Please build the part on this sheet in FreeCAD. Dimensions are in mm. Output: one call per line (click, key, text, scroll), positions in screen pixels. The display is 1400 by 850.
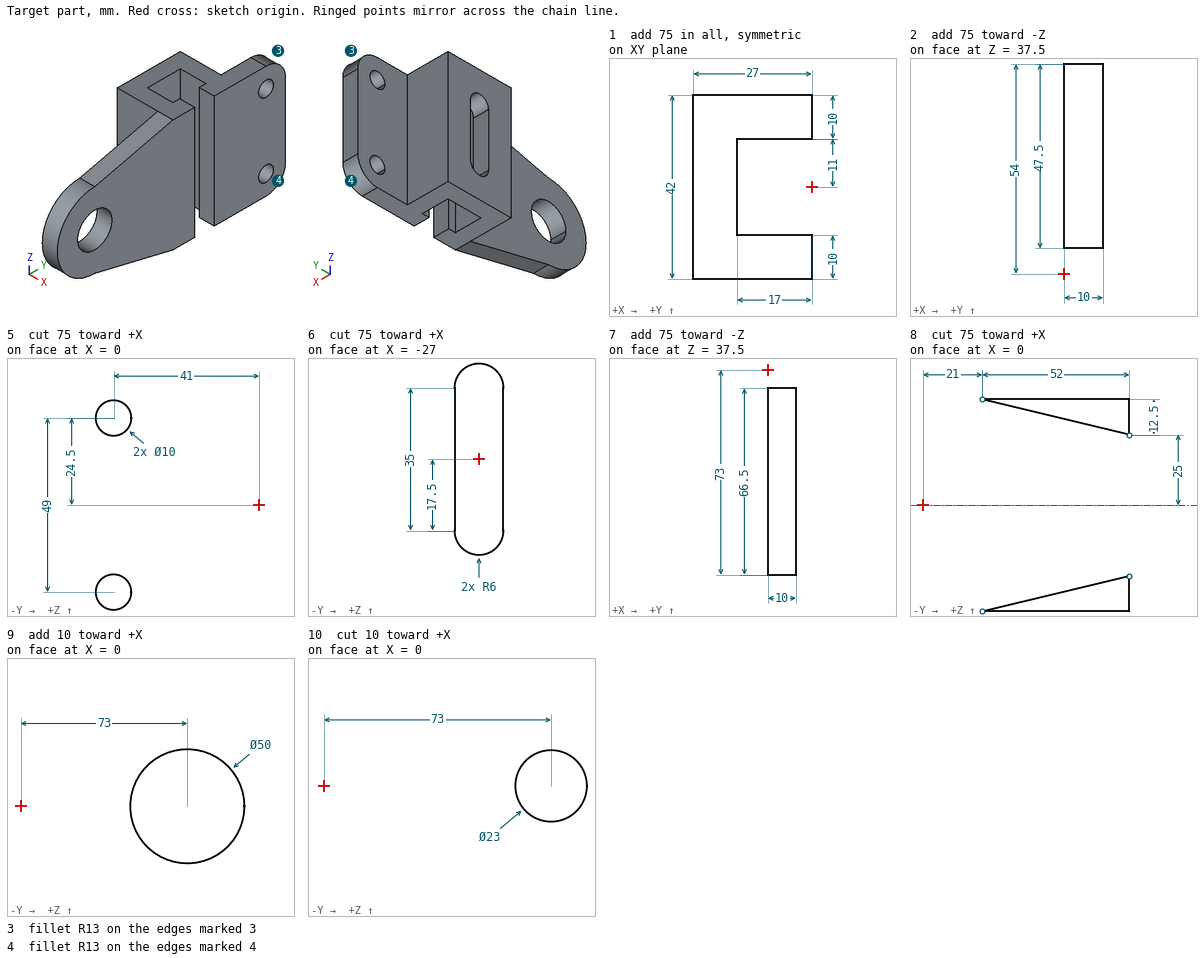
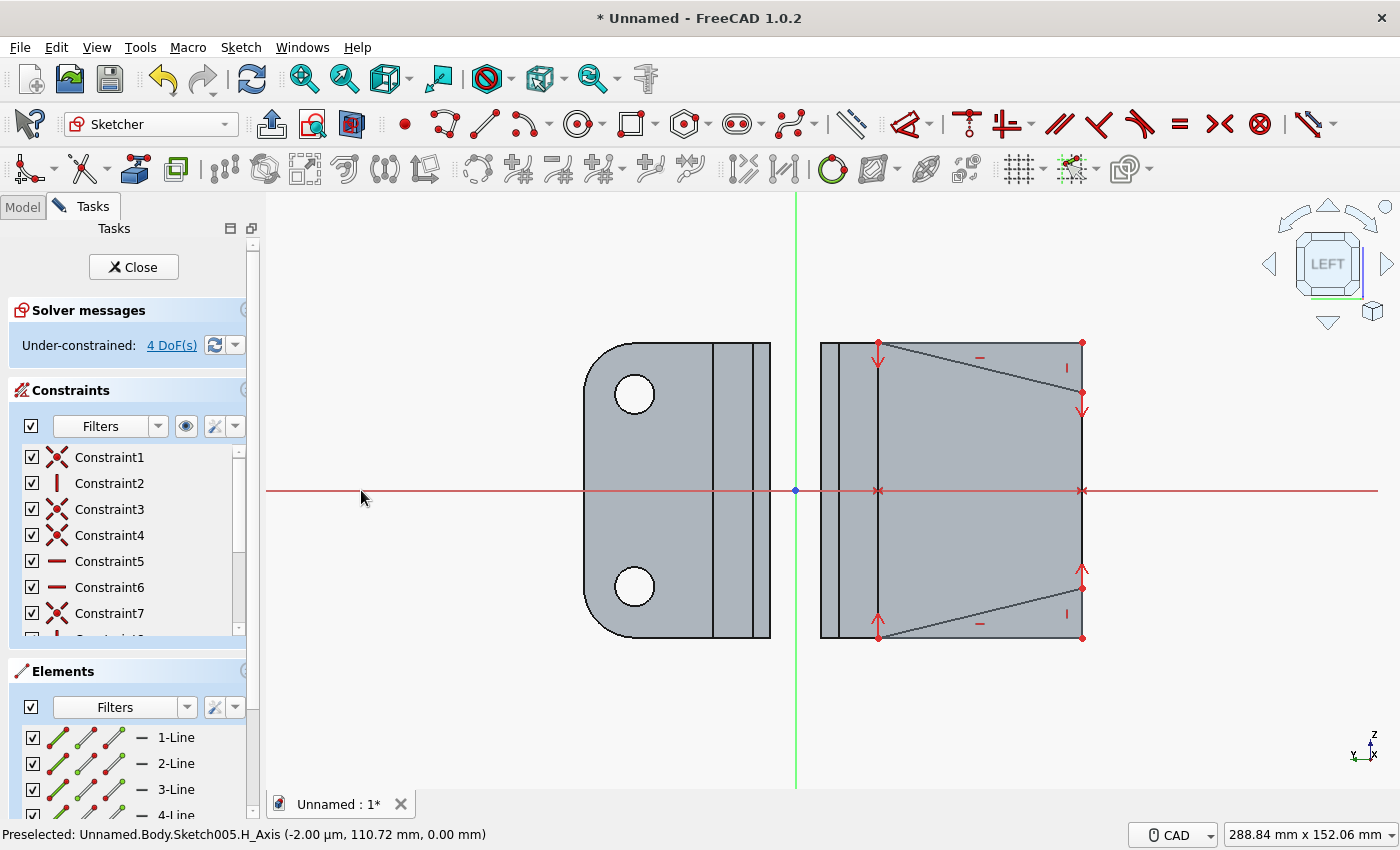
click(1021, 343)
click(980, 309)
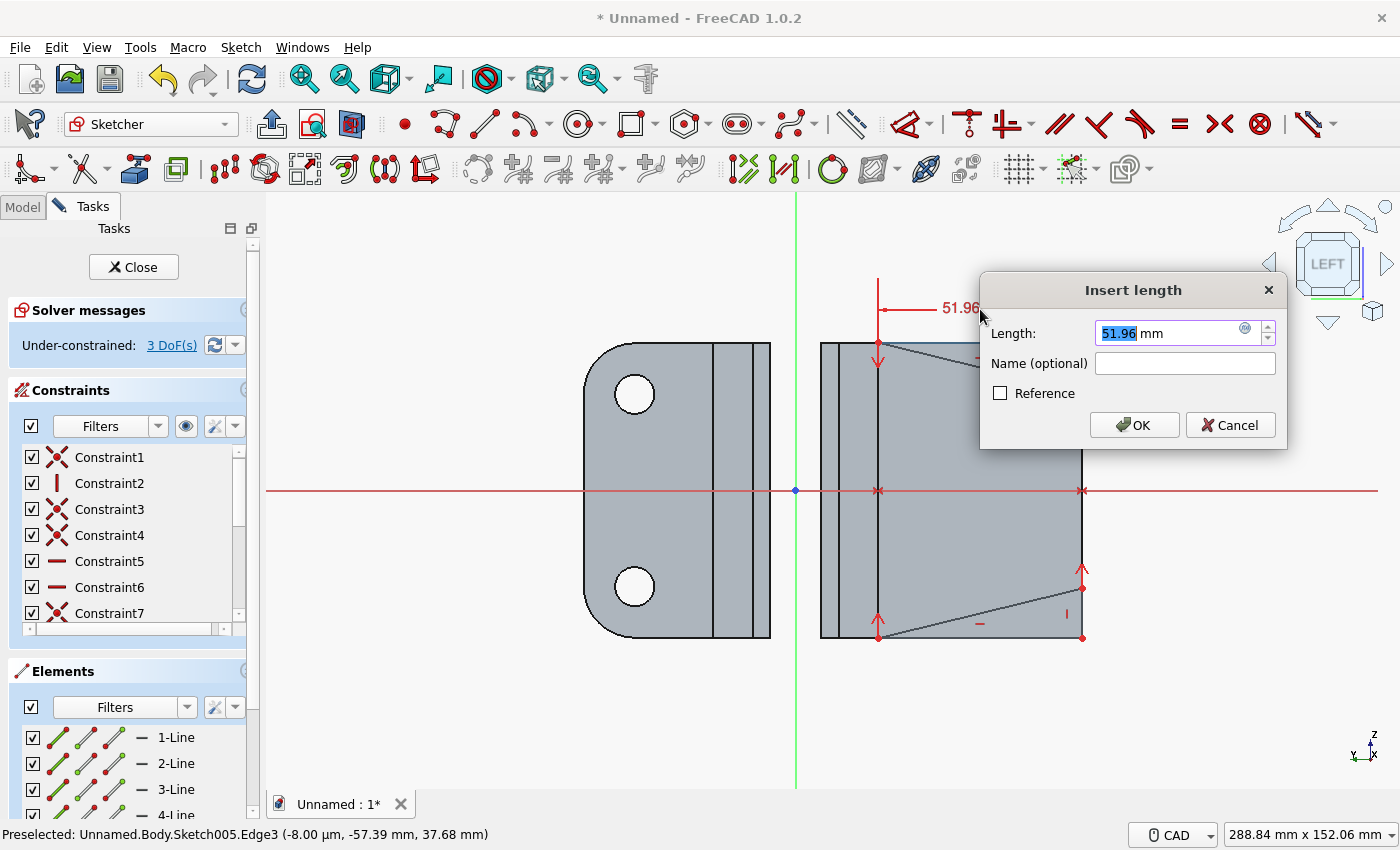
text(52)
key(Return)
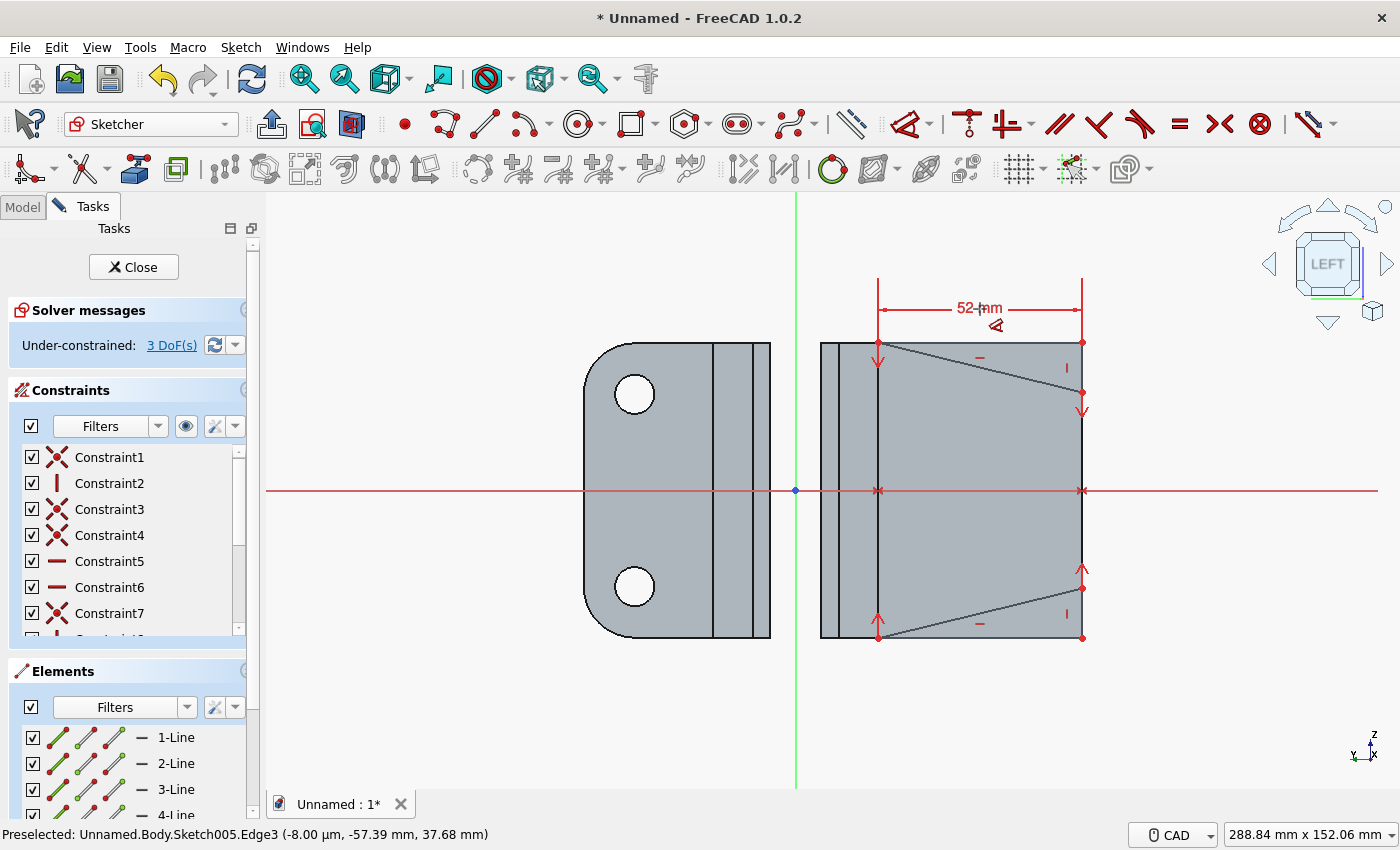
click(878, 343)
click(837, 309)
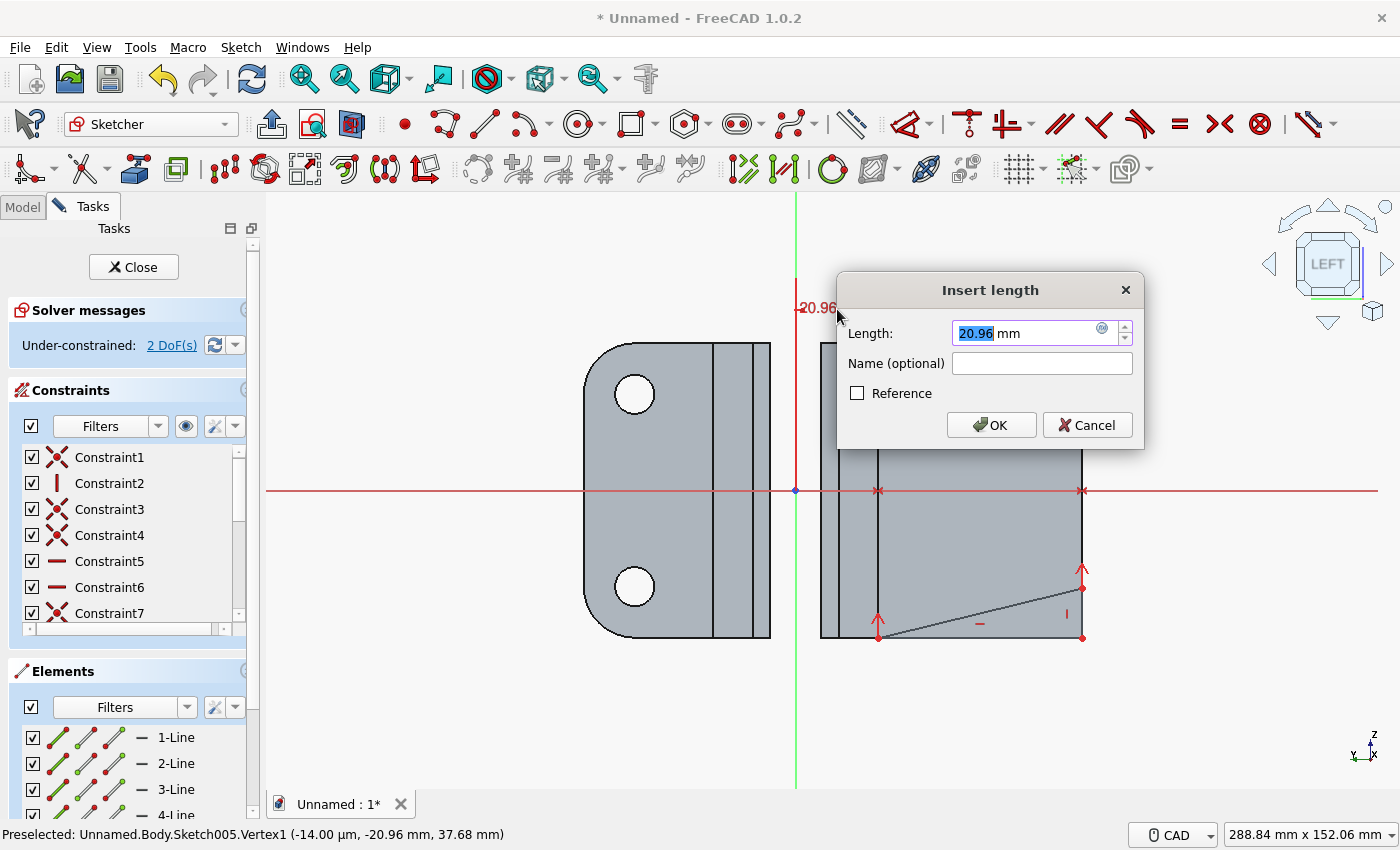
text(21)
key(Return)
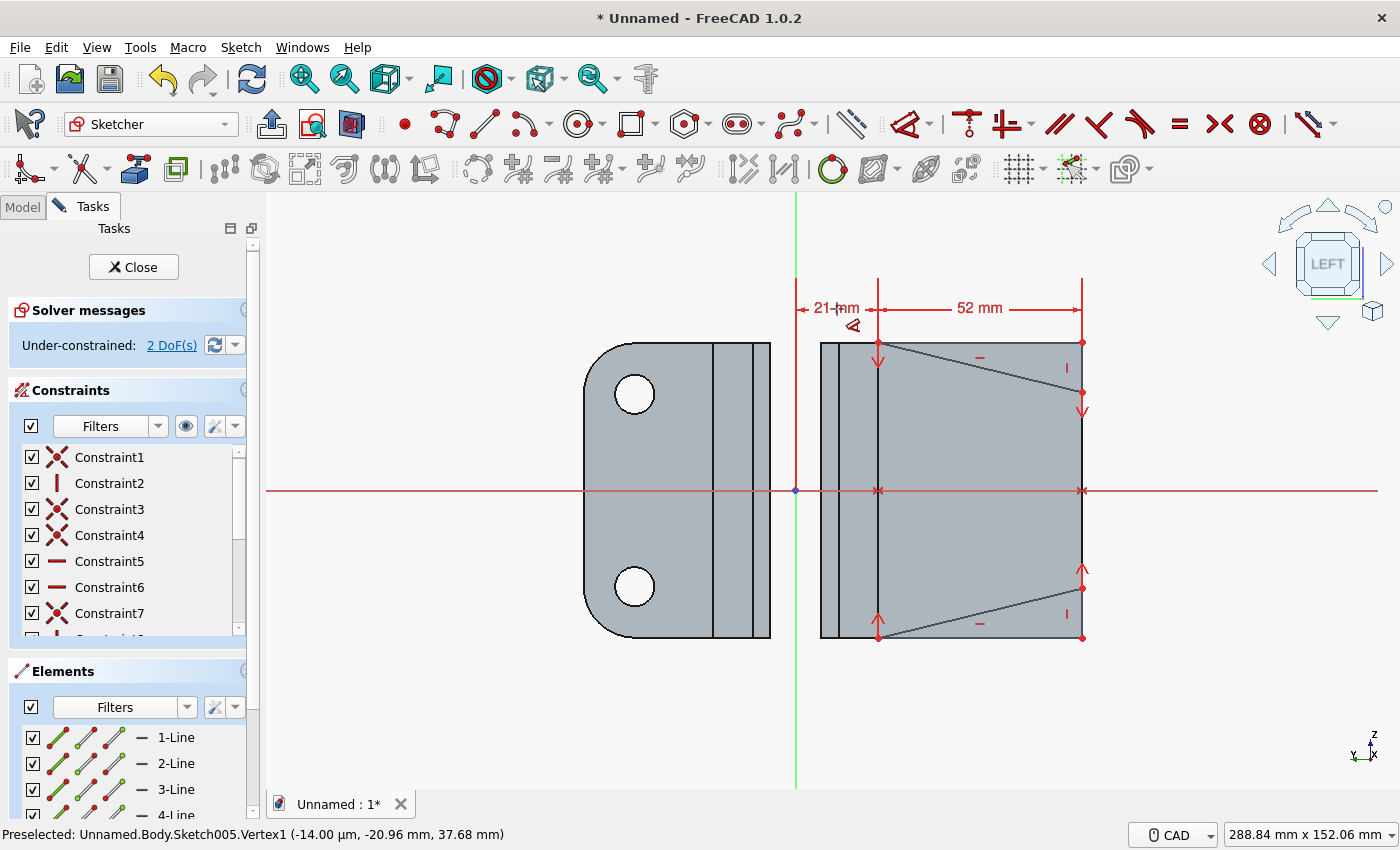
click(1082, 392)
click(1116, 441)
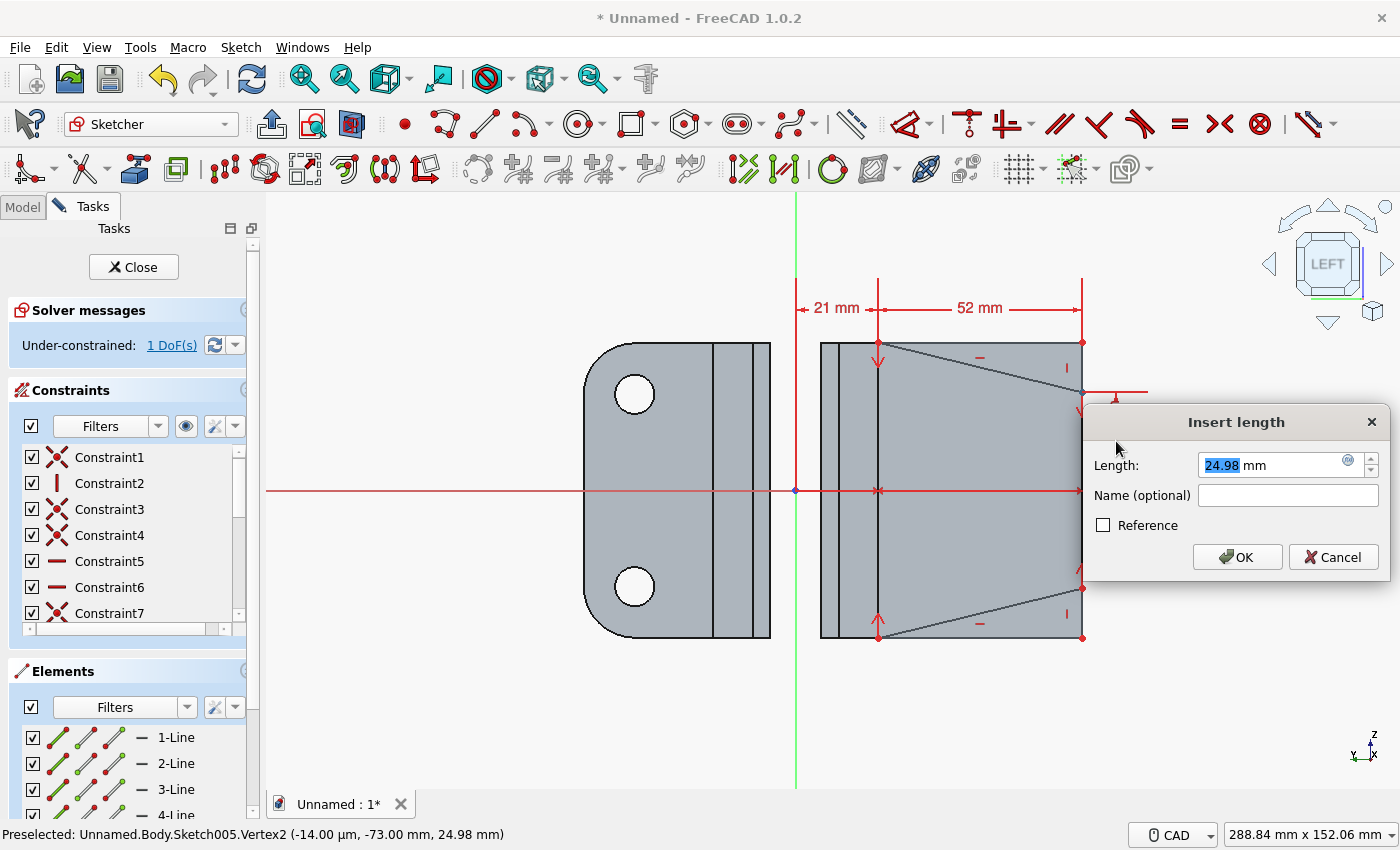
text(25)
key(Return)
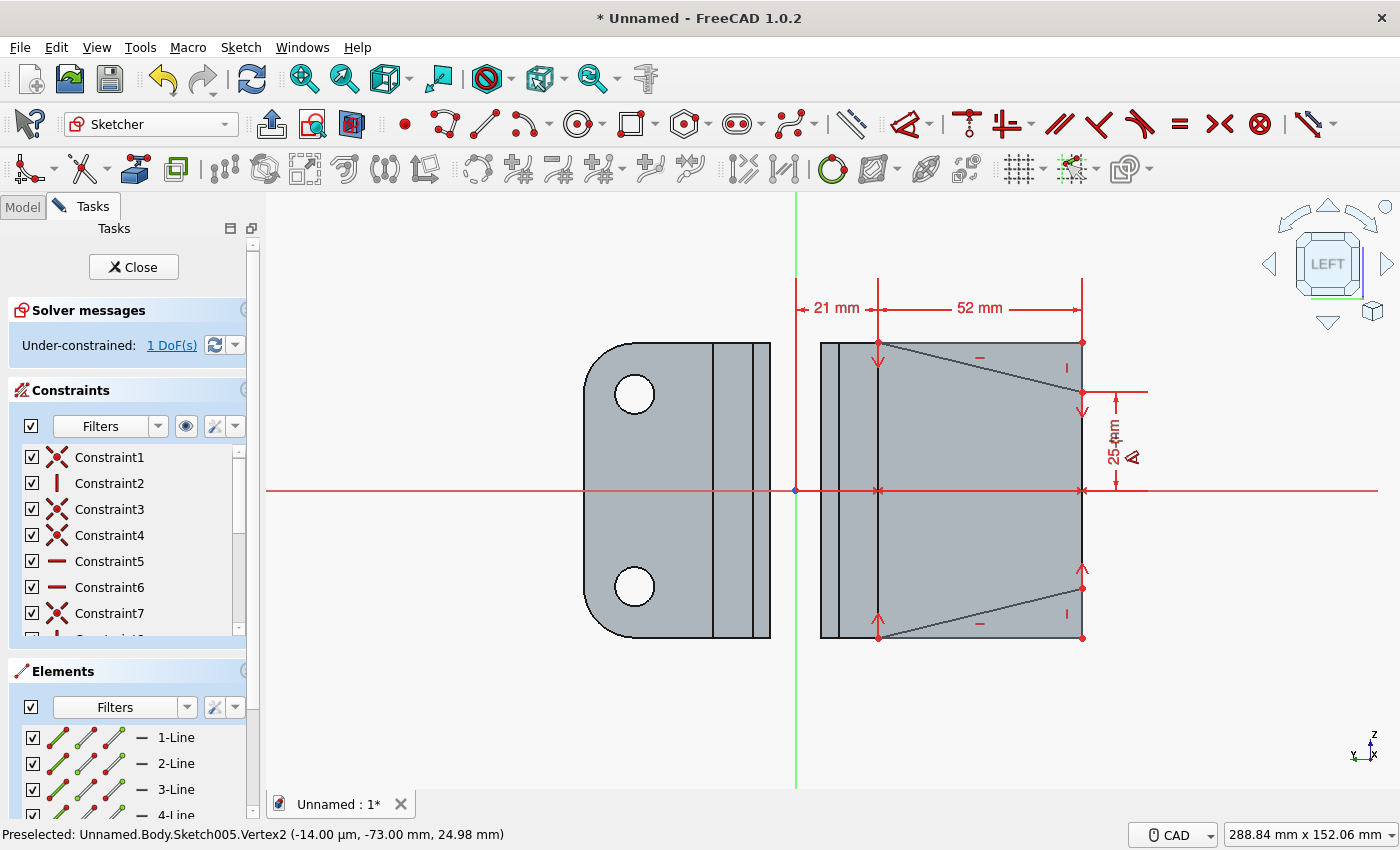
click(1082, 377)
click(1116, 367)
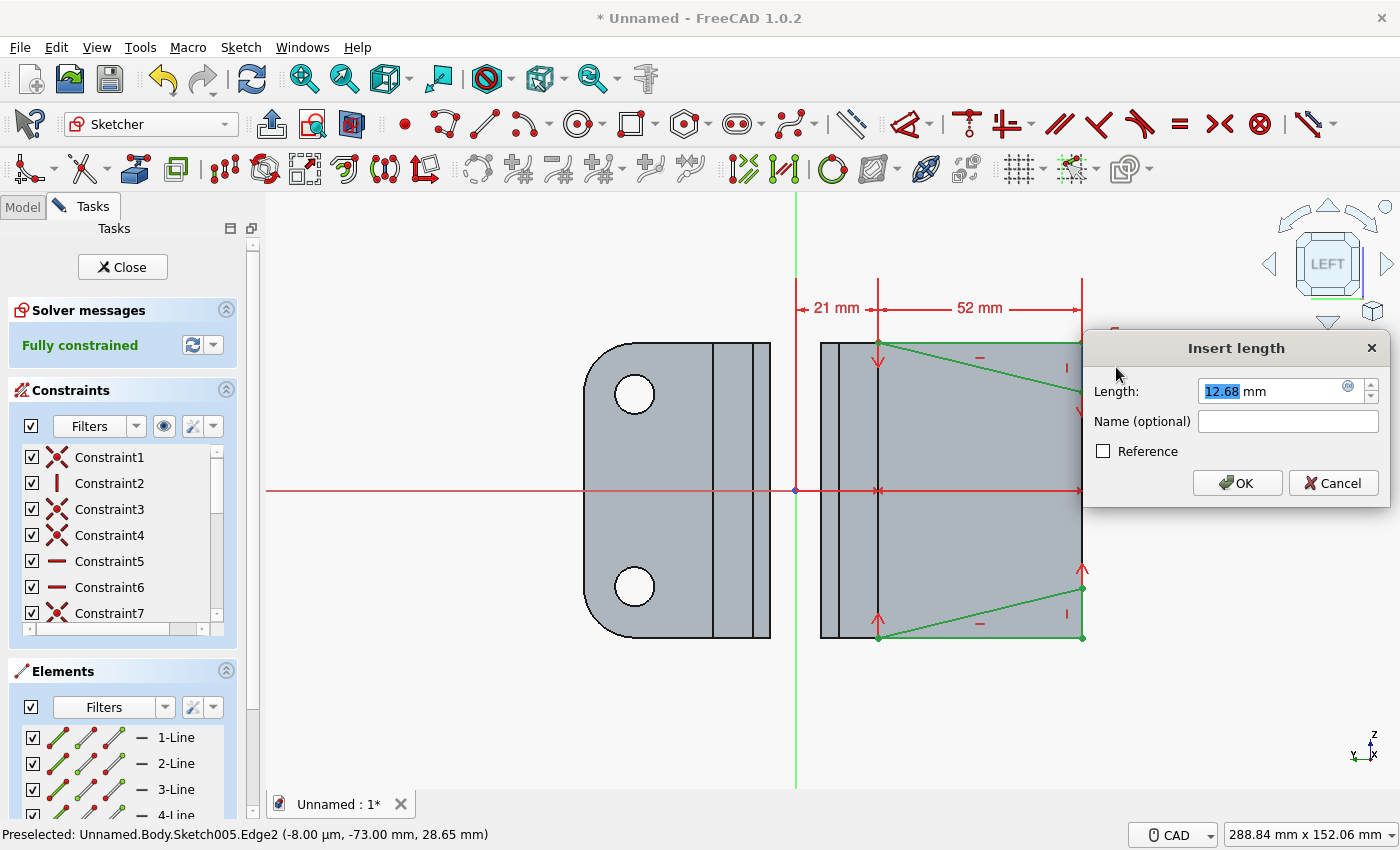
text(12.5)
key(Return)
key(Escape)